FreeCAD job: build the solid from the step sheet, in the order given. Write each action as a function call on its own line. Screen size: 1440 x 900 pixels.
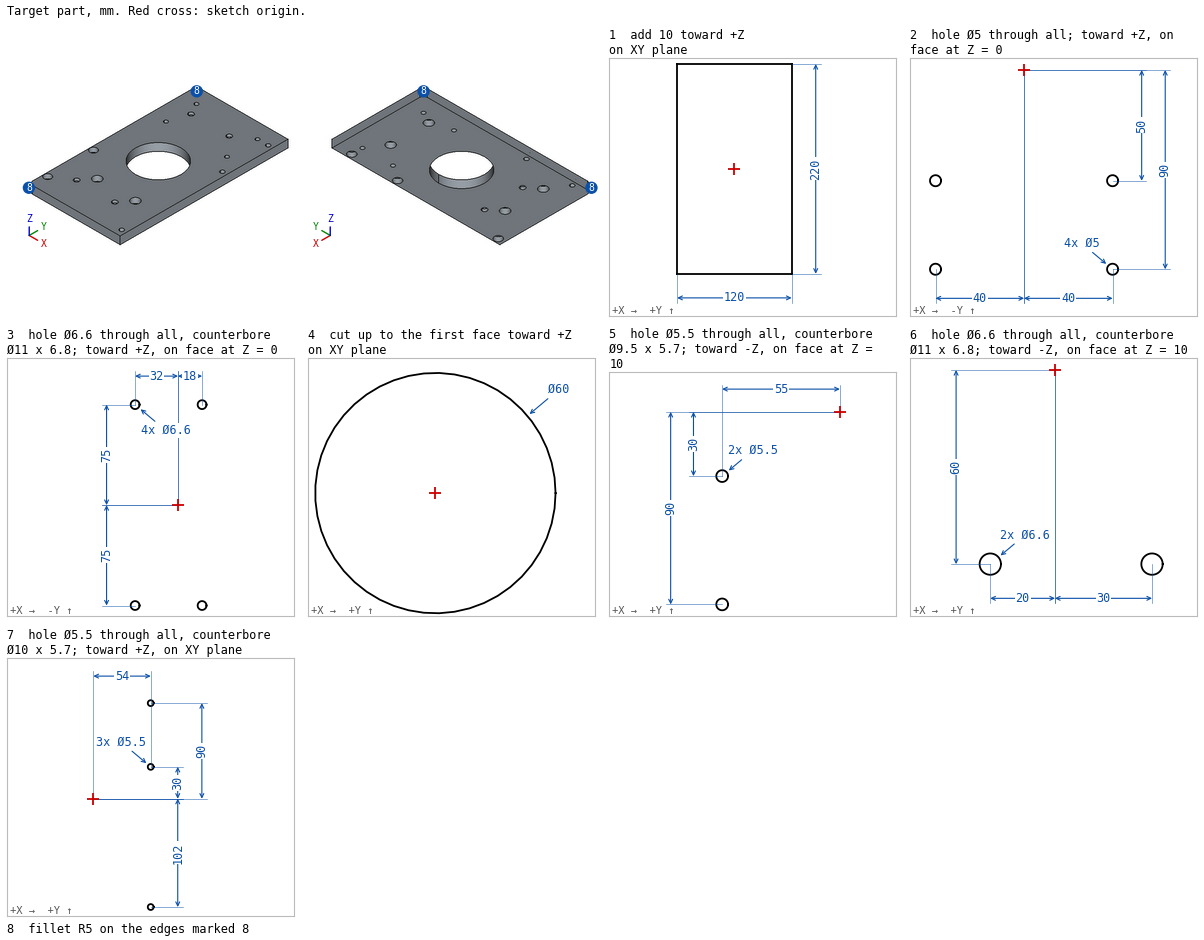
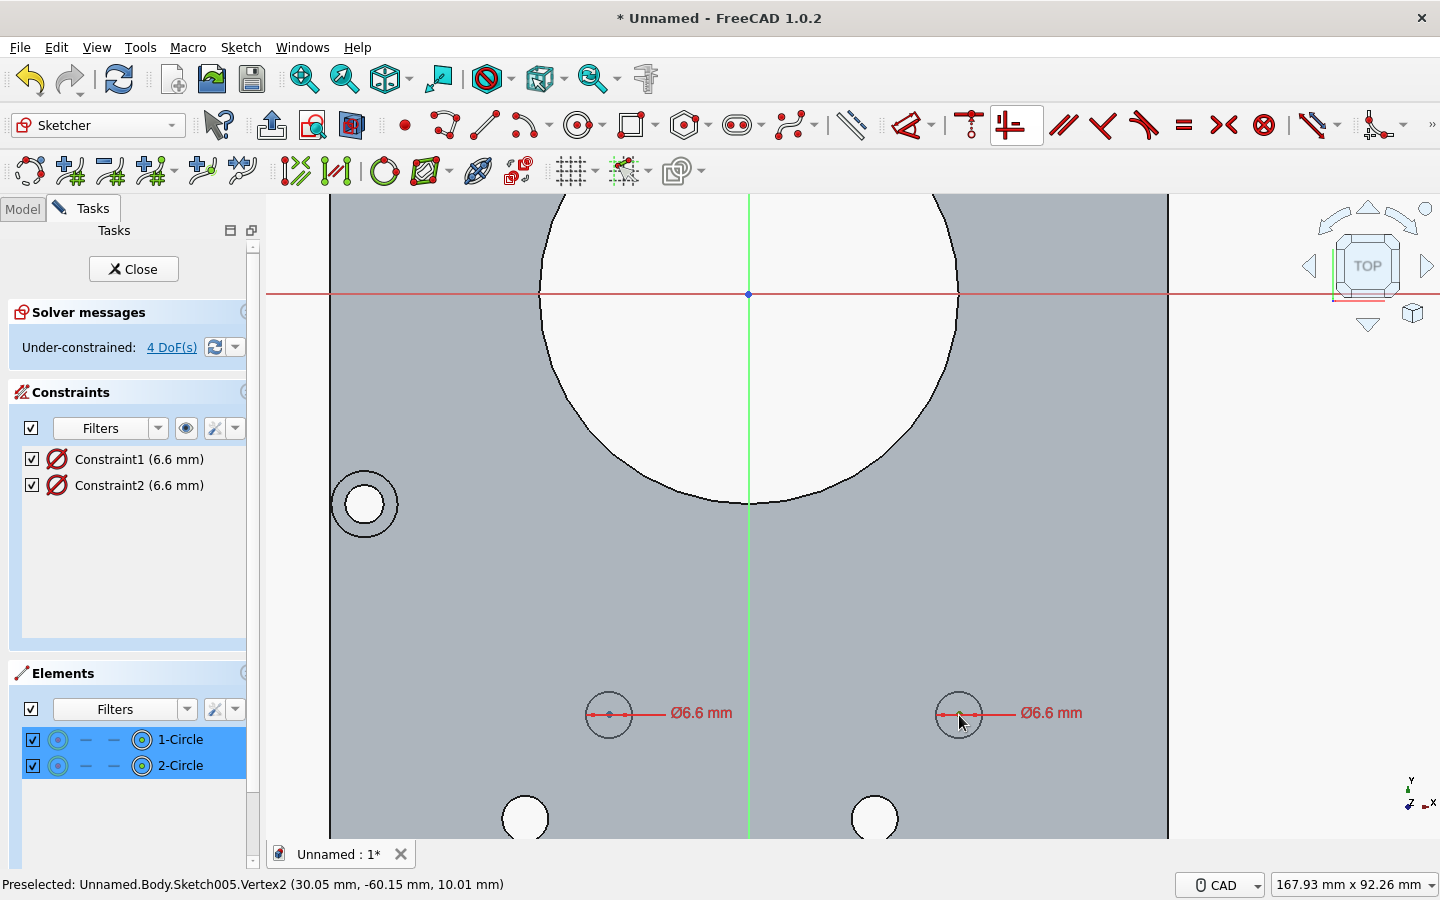
key(h)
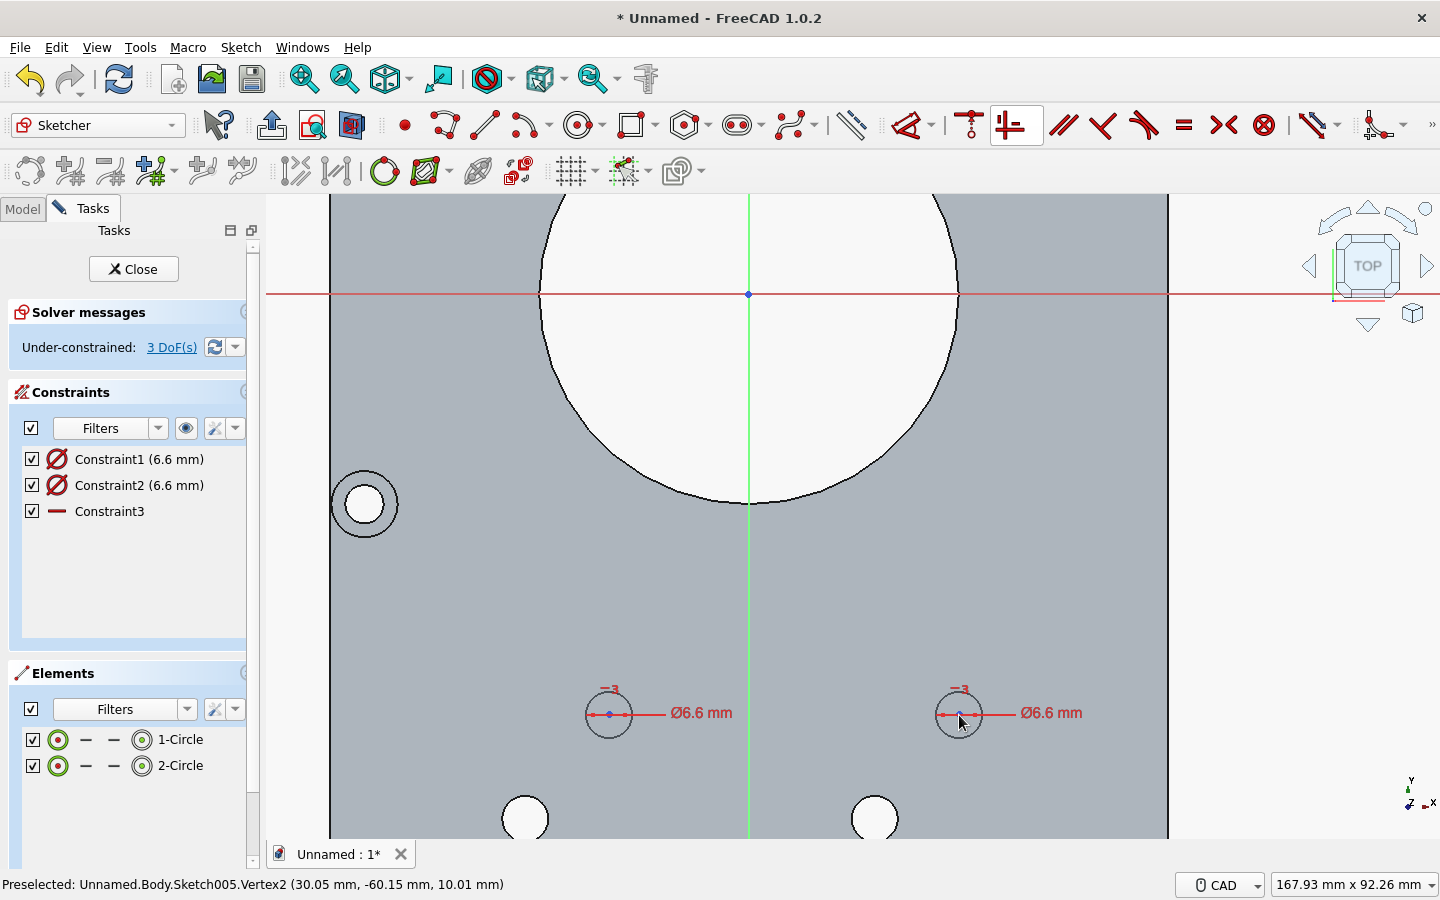
click(906, 126)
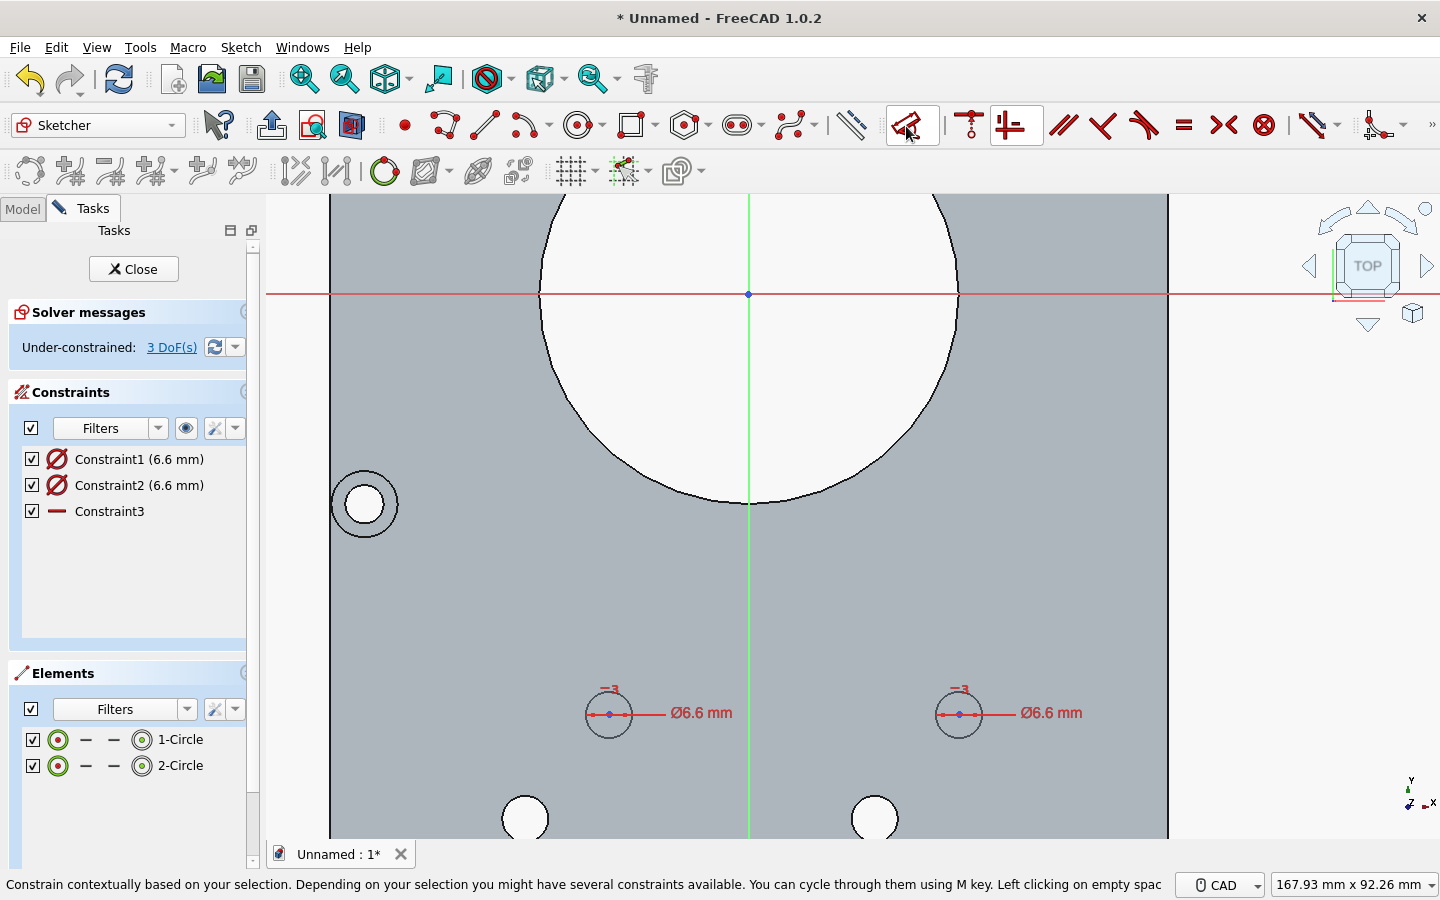
click(609, 715)
click(679, 260)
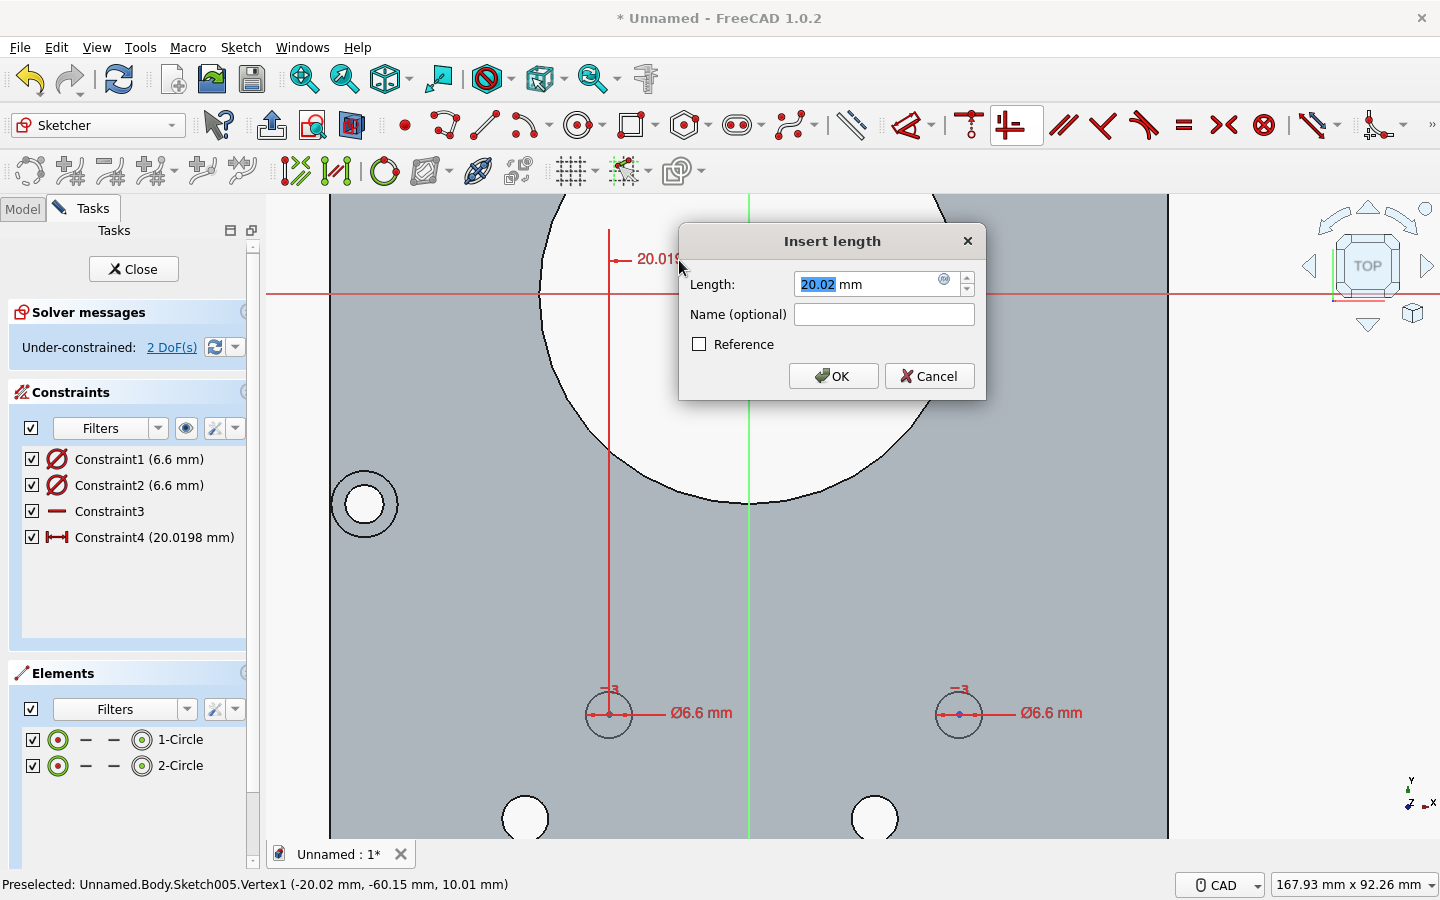
text(20)
key(Return)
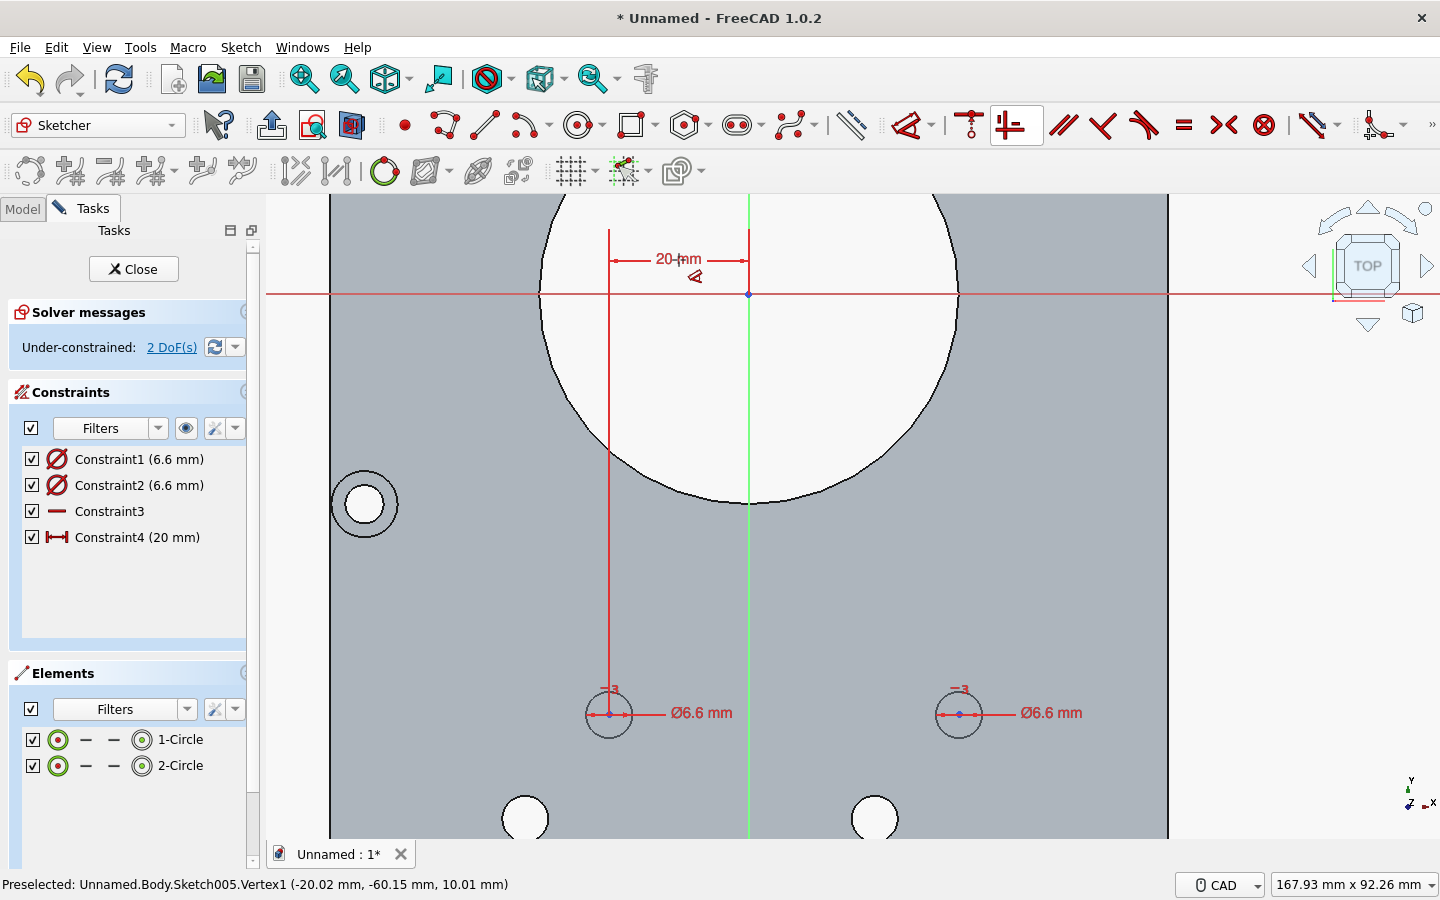
click(609, 715)
click(575, 505)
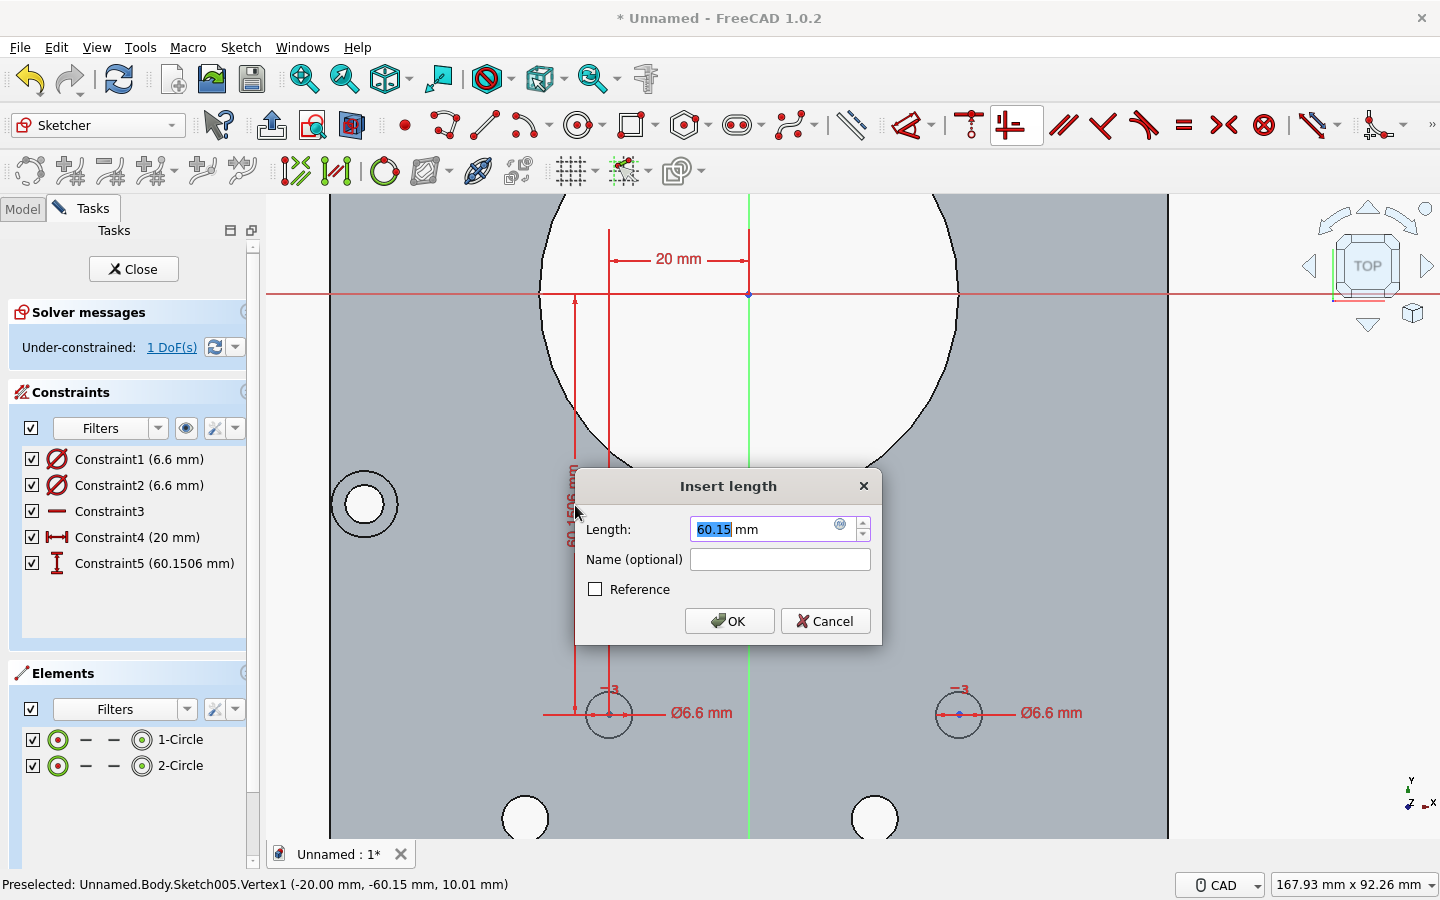
text(60)
key(Return)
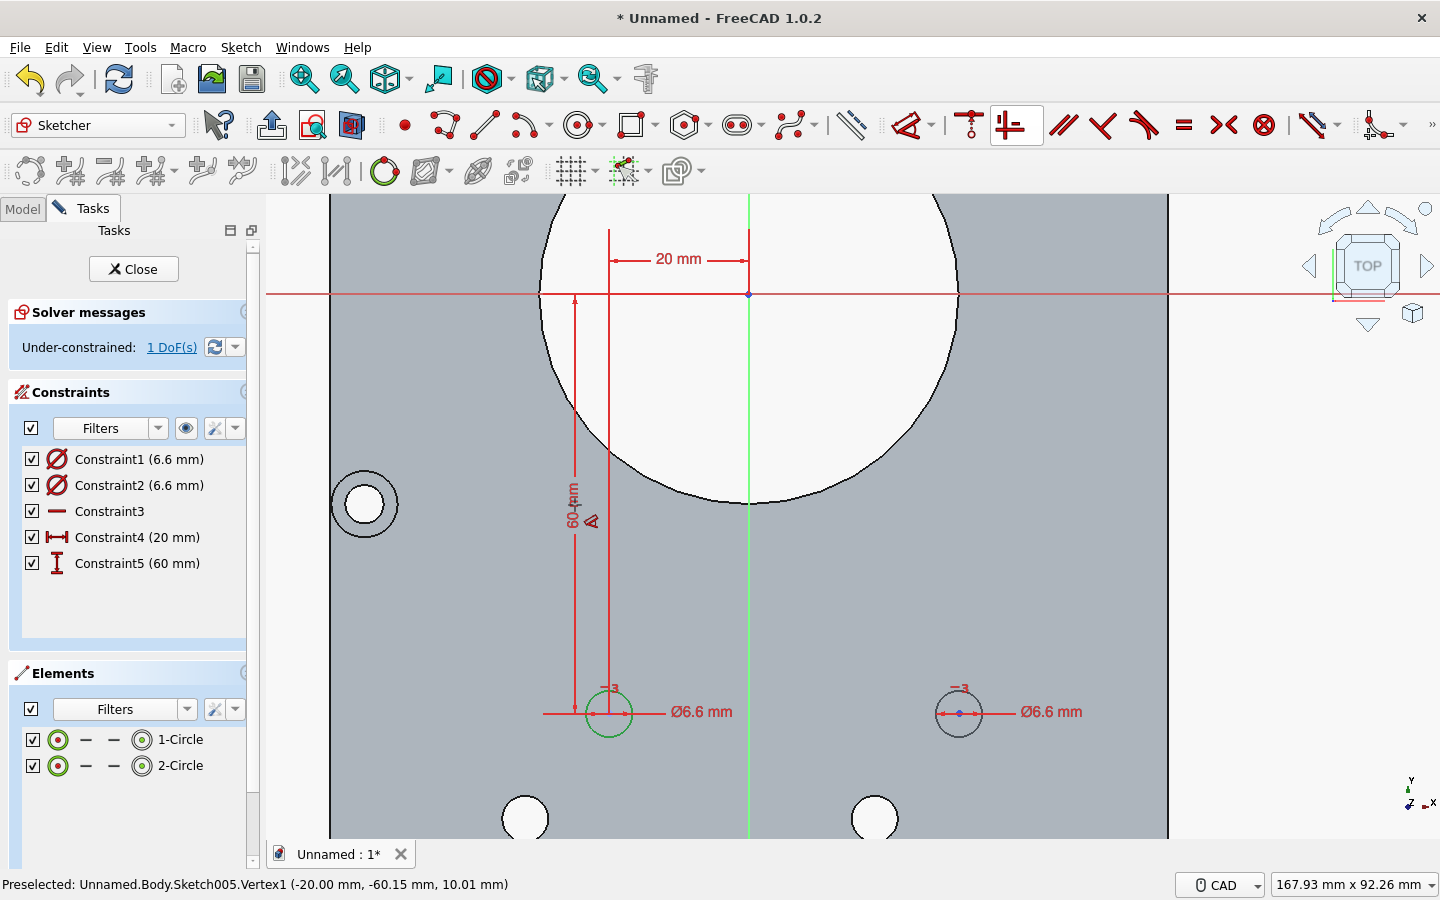
click(959, 714)
click(854, 260)